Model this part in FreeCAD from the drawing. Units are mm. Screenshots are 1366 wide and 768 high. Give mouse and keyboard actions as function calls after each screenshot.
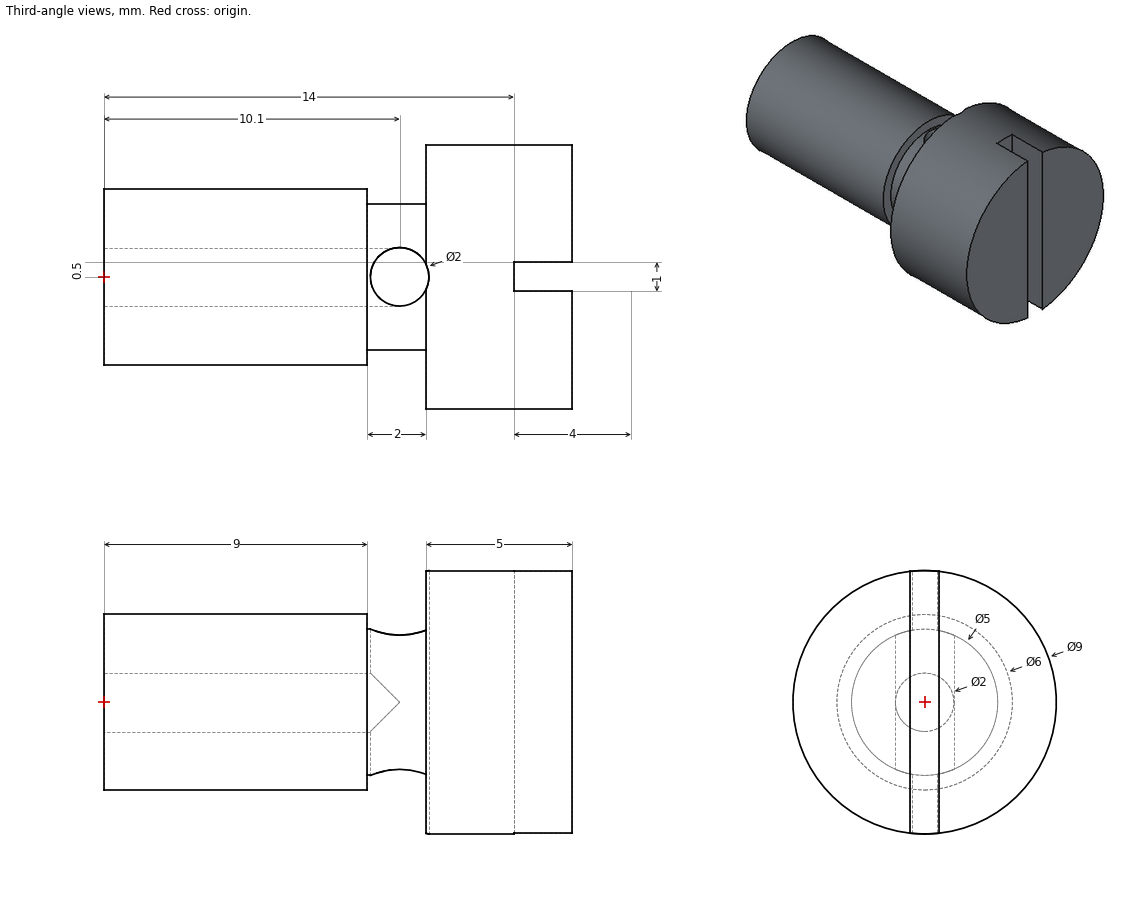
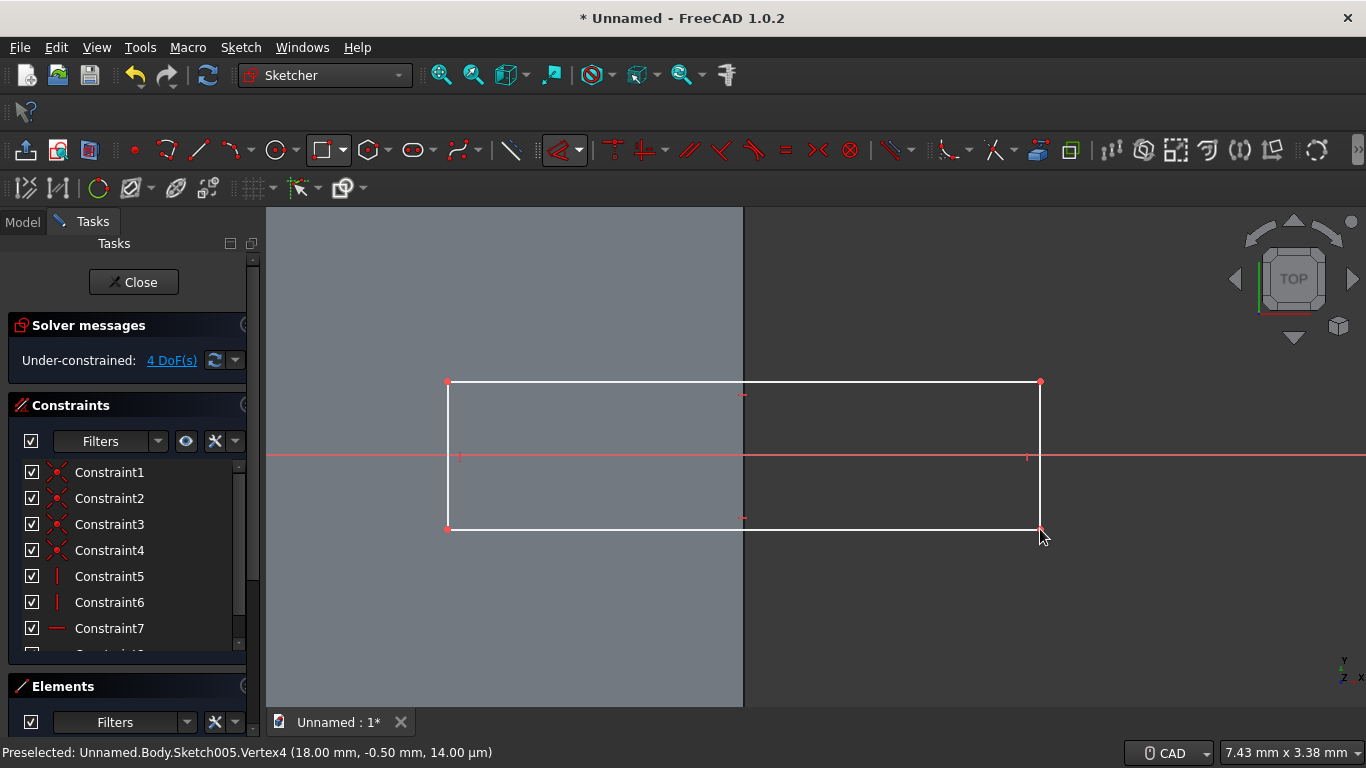
click(448, 426)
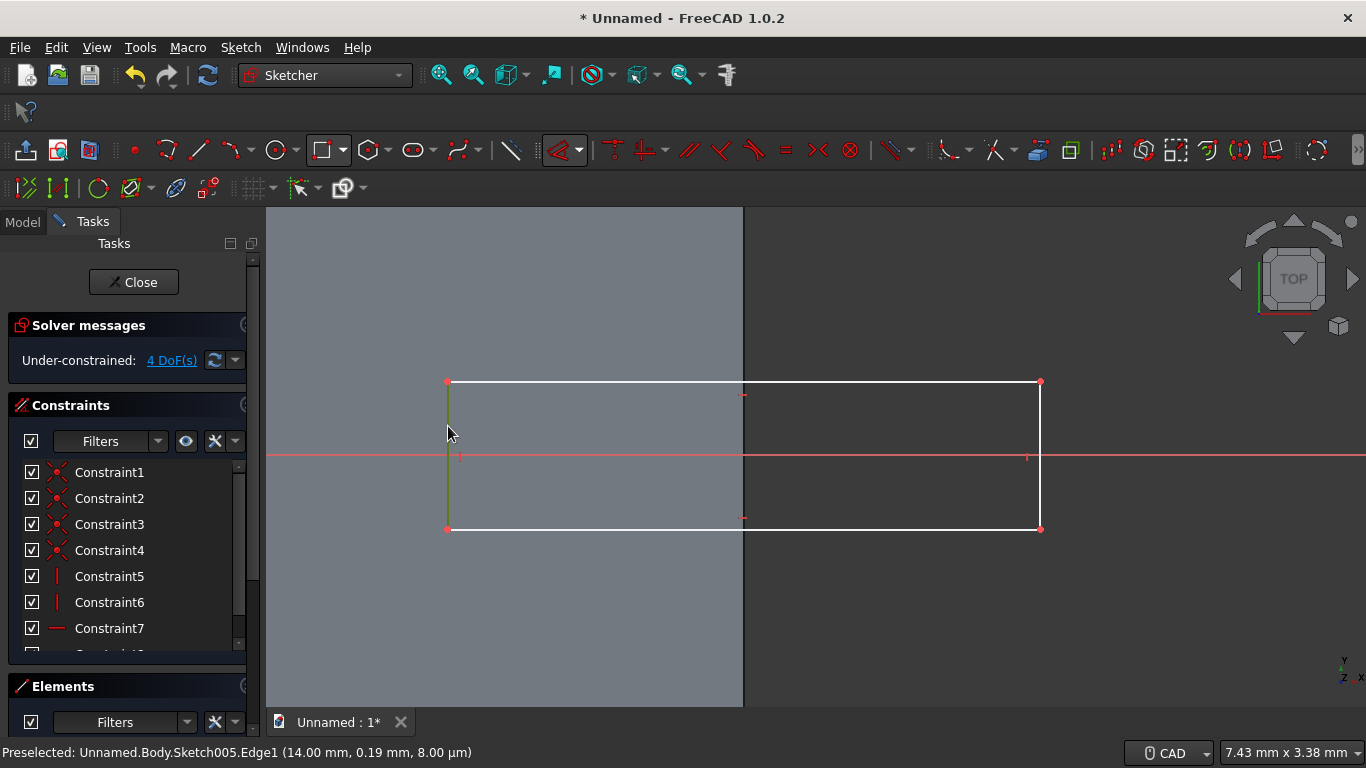
key(i)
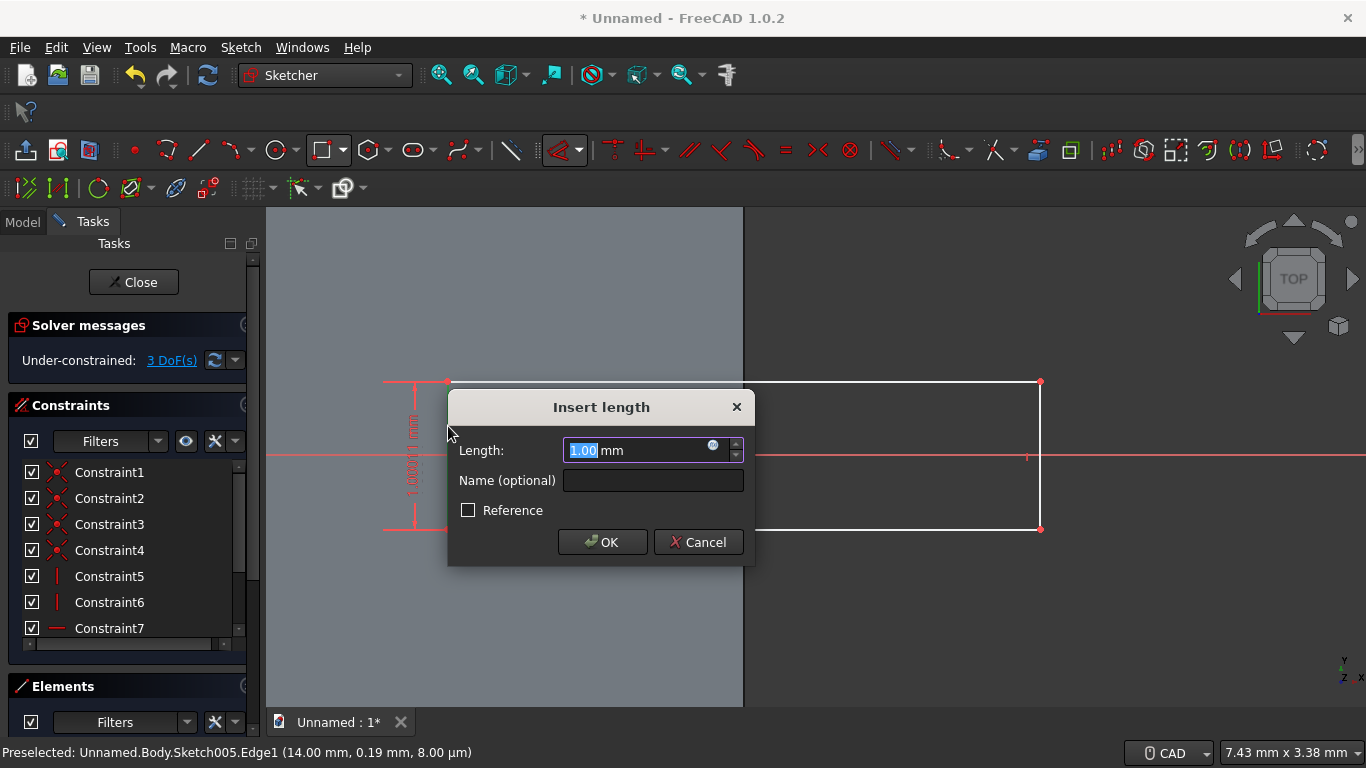
text(1)
key(Return)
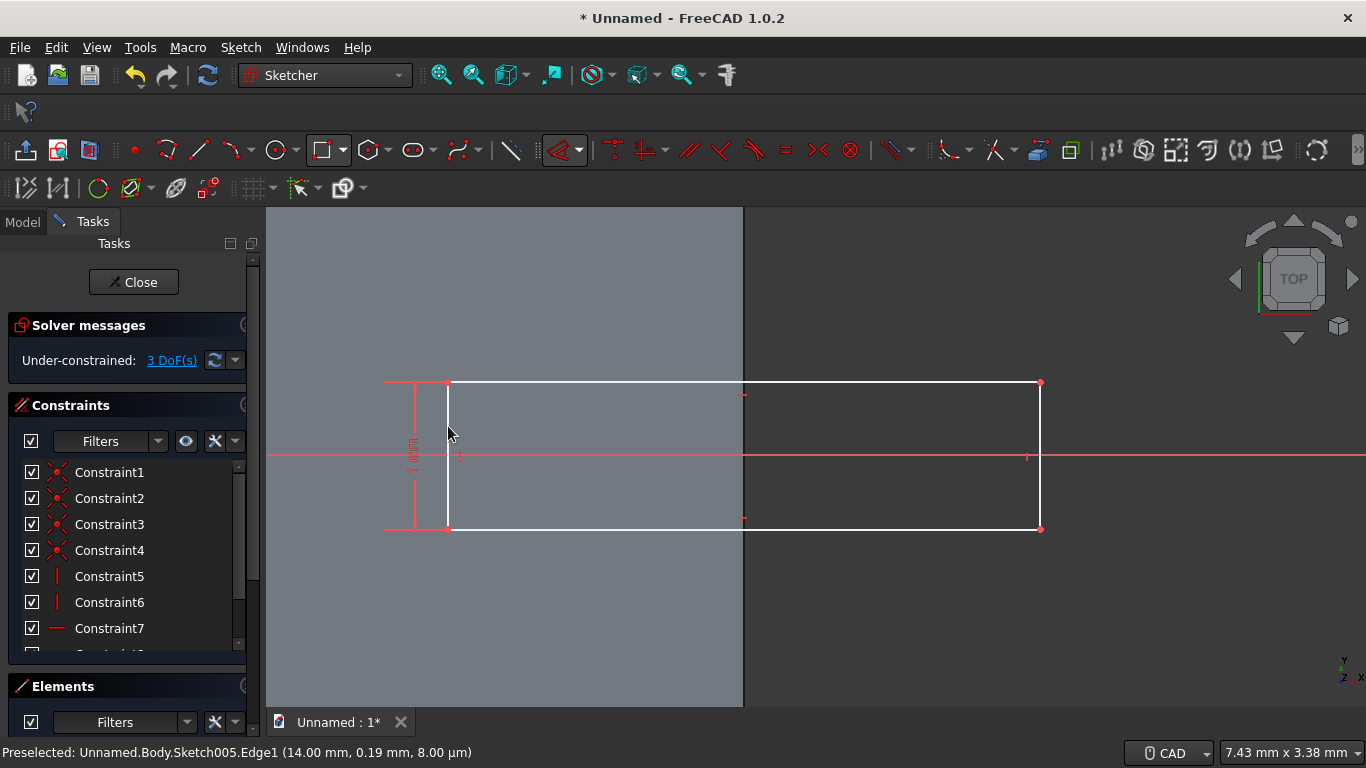
click(626, 530)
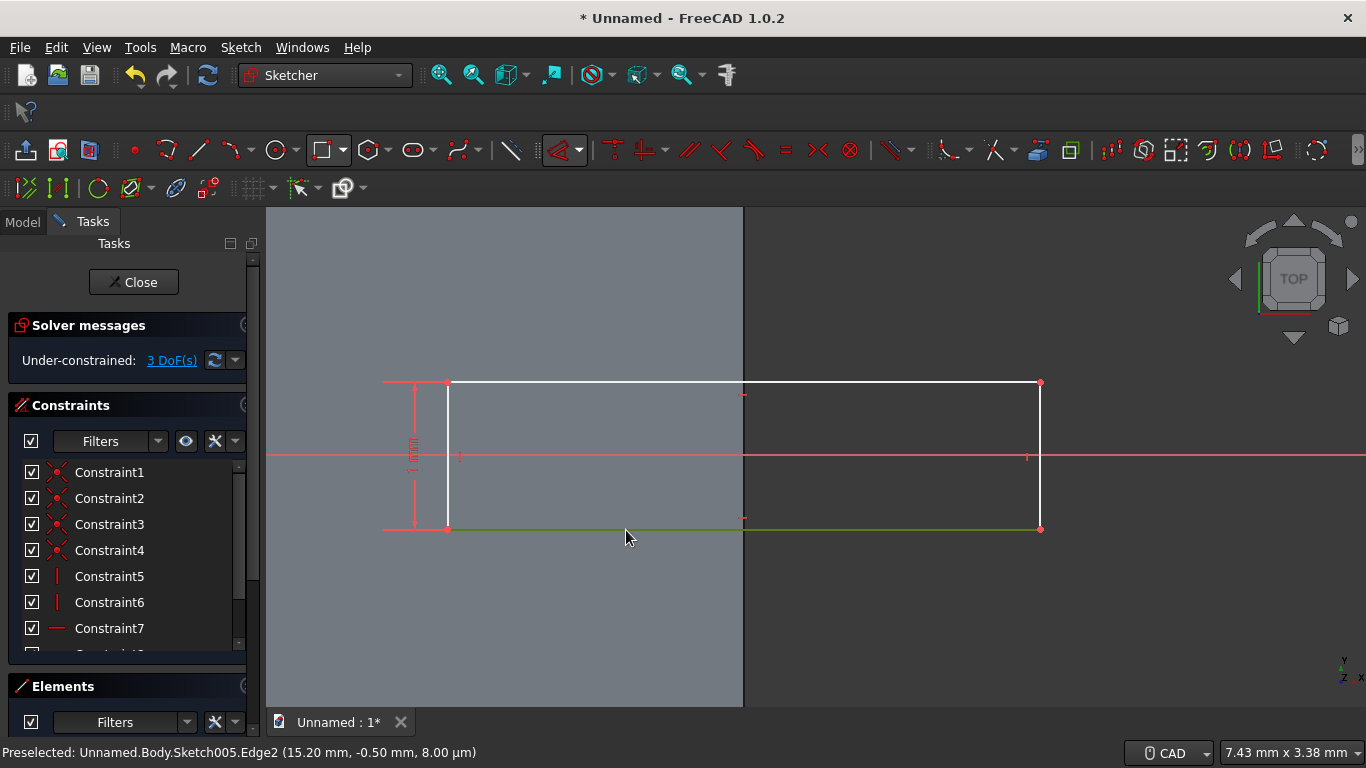
click(582, 150)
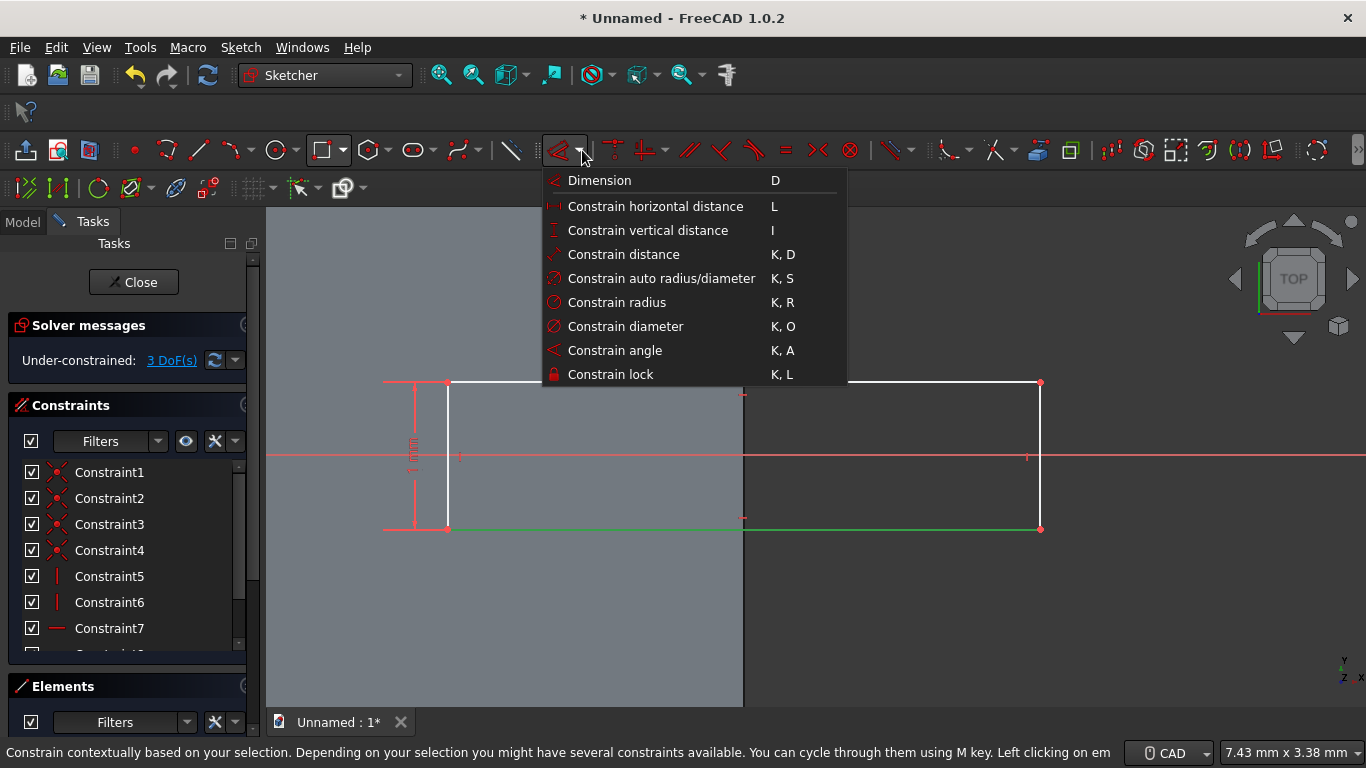
click(695, 206)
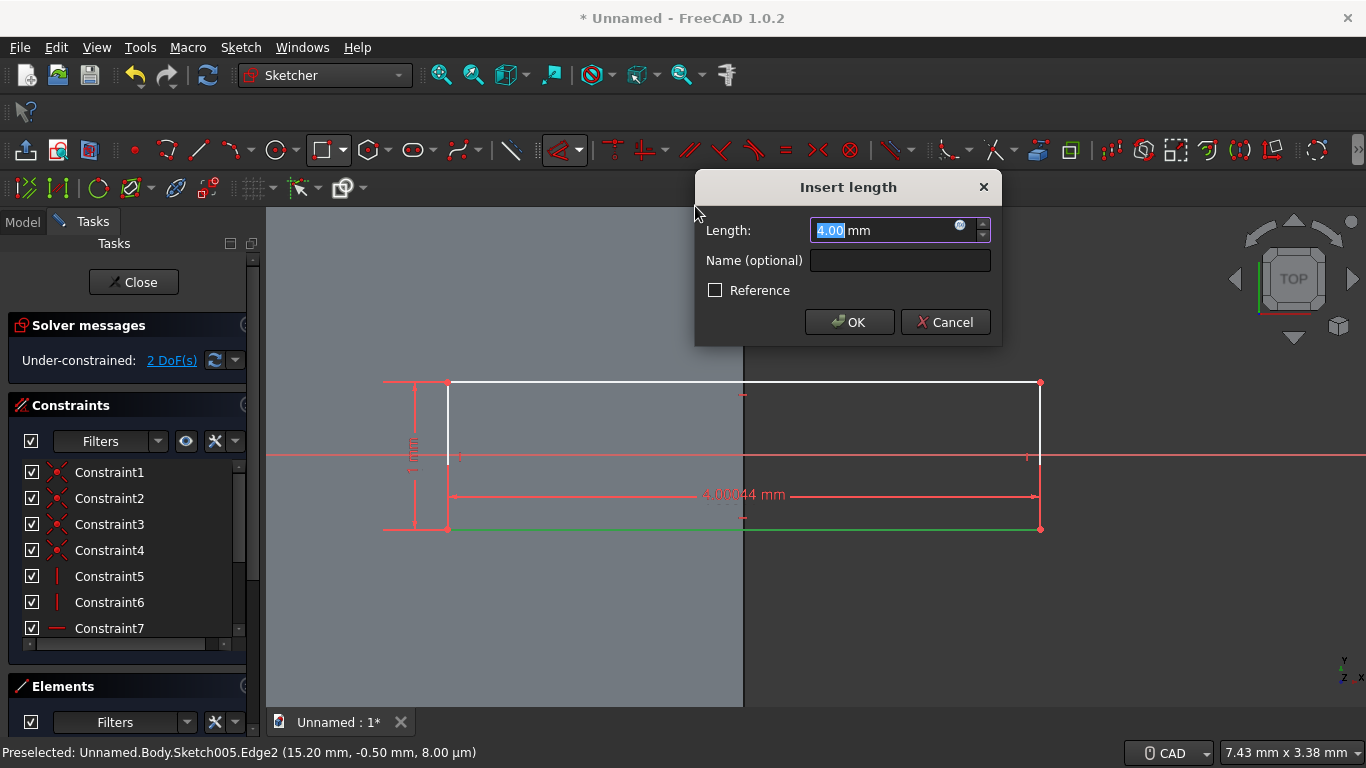
text(4)
key(Return)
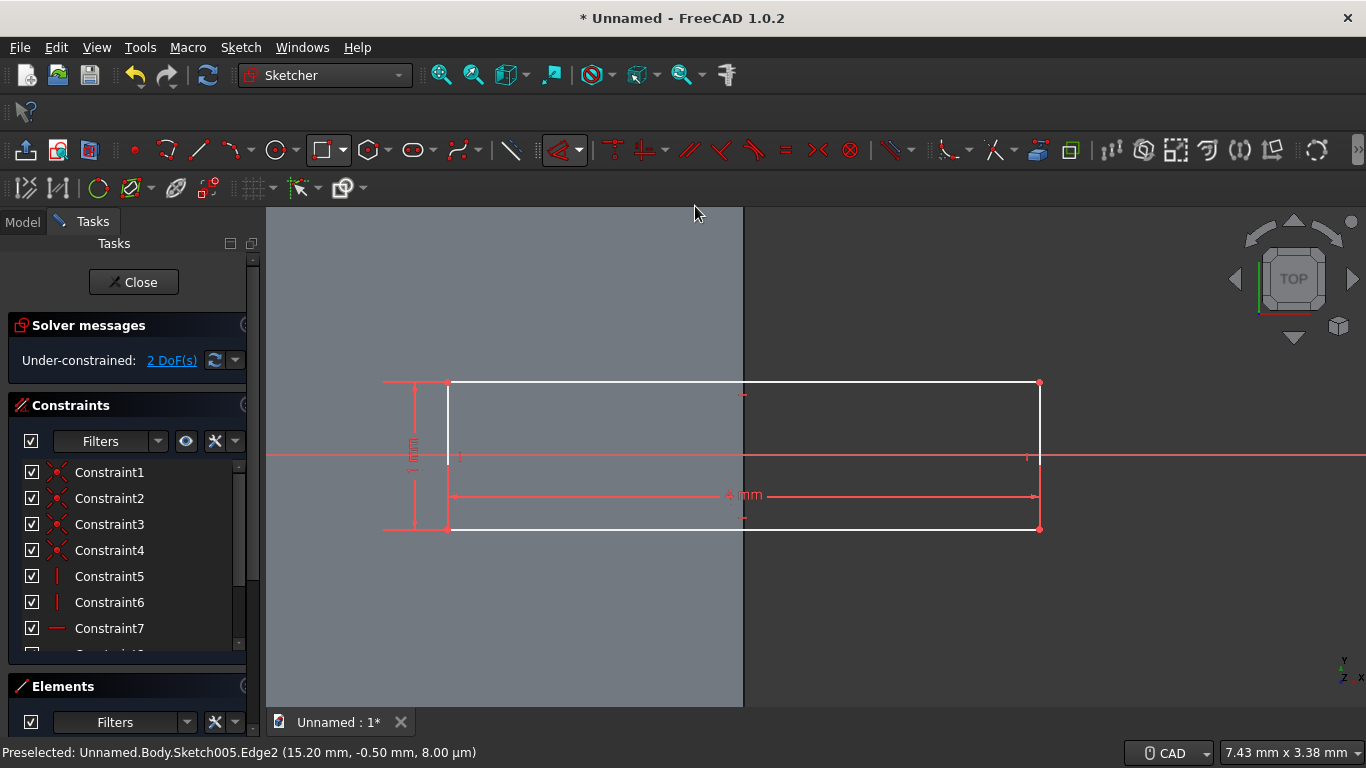
click(448, 382)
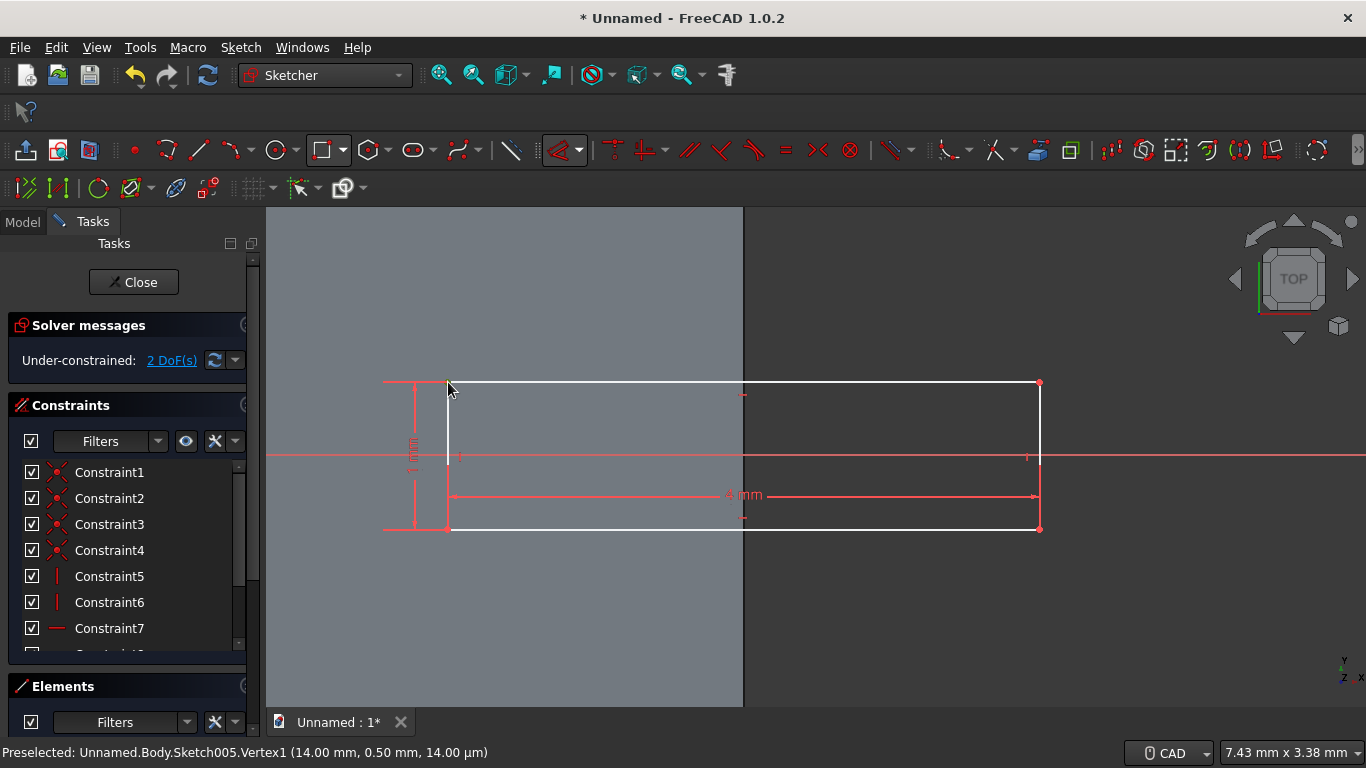
key(l)